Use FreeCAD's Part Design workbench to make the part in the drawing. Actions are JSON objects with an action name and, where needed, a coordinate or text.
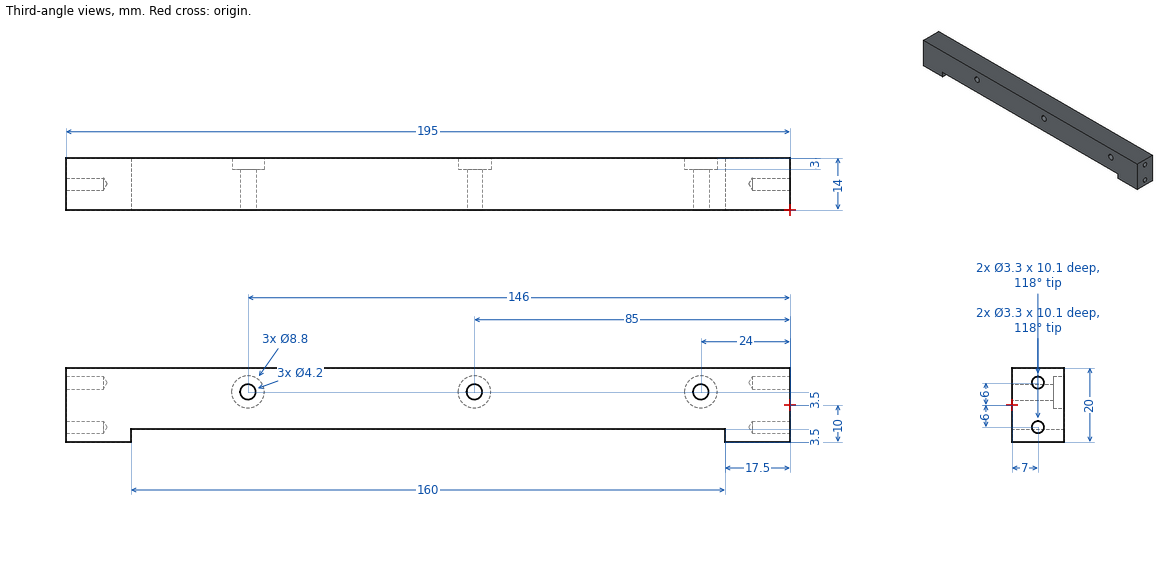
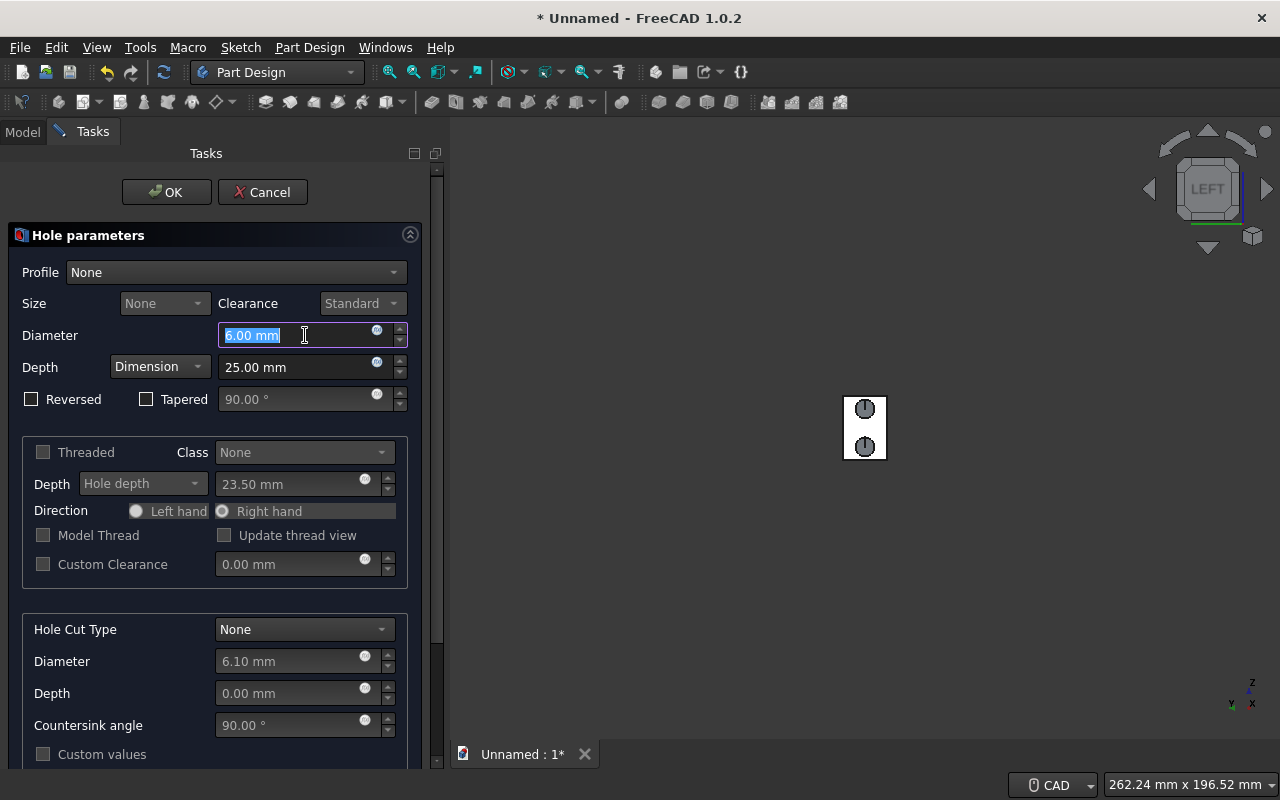
{"action": "type", "text": "3.3"}
{"action": "key", "text": "Tab"}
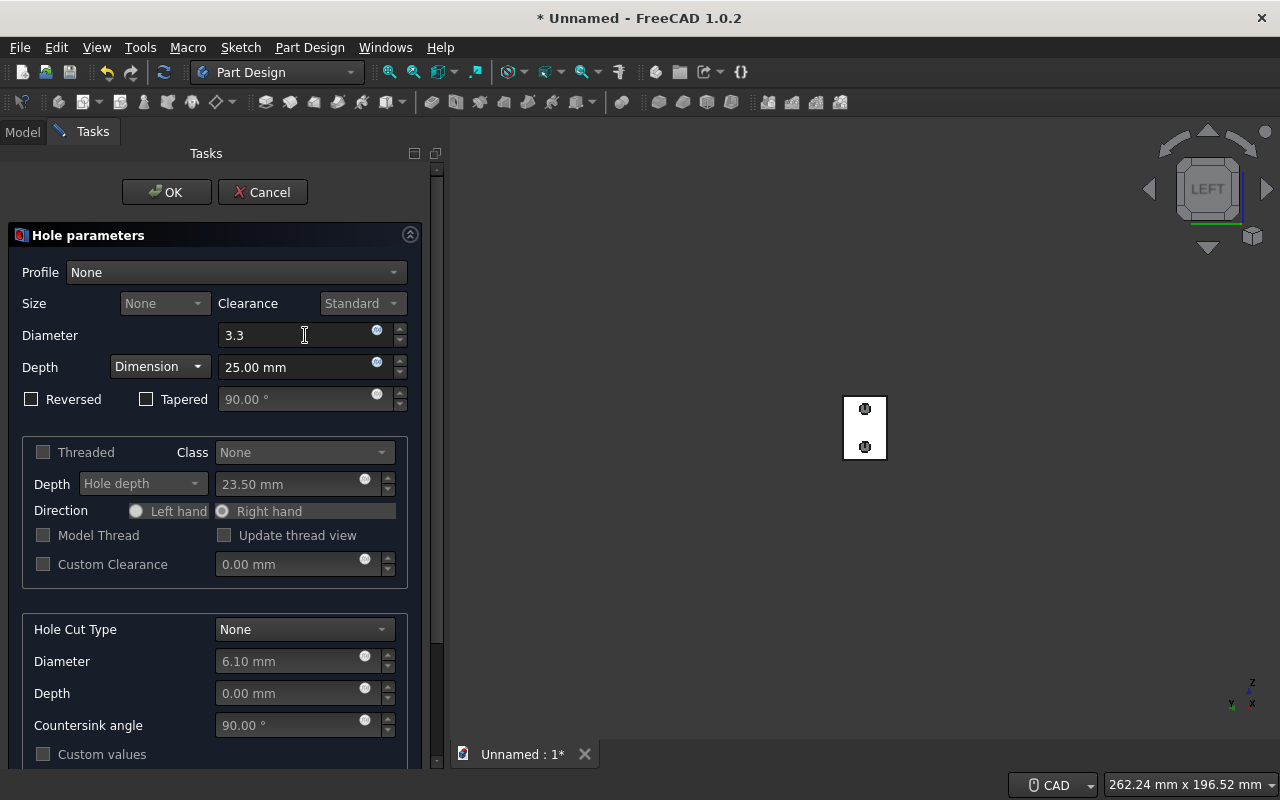
{"action": "triple_click", "coordinate": [305, 367]}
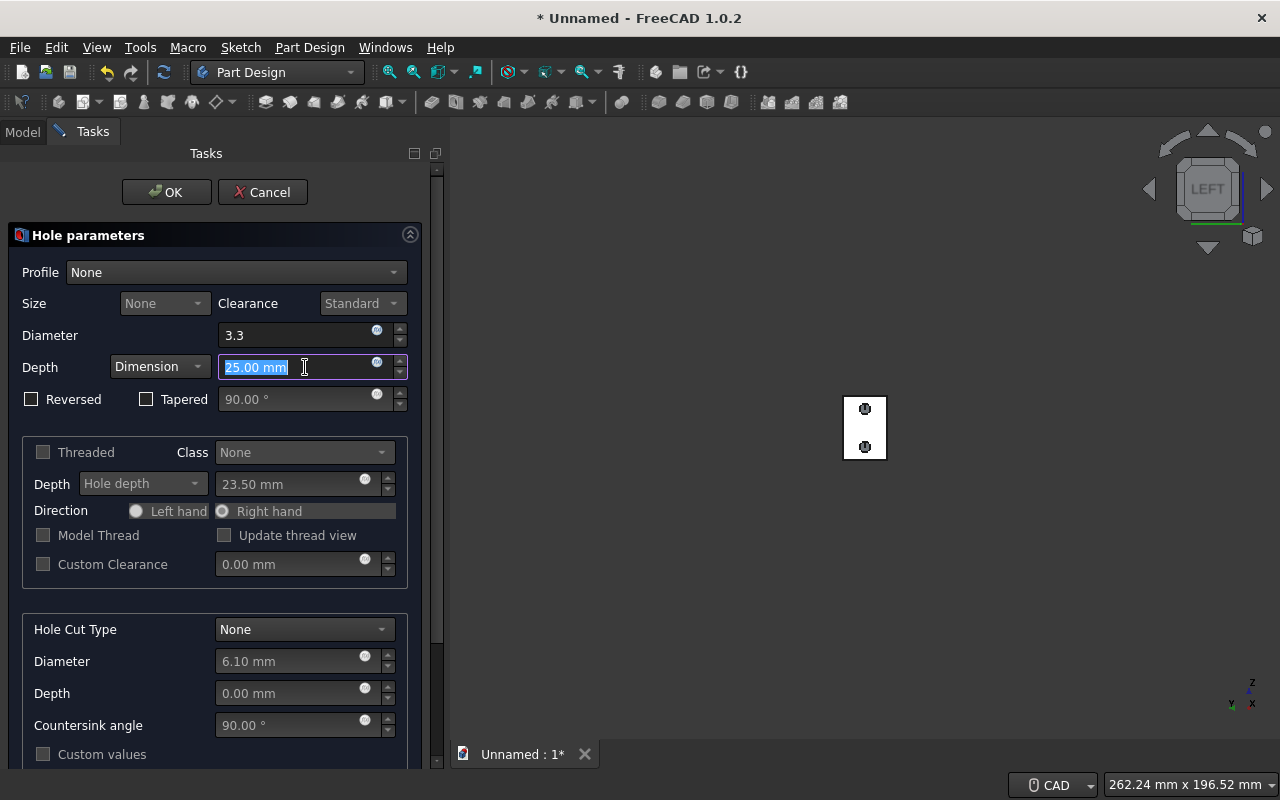
{"action": "type", "text": "10.1"}
{"action": "key", "text": "Tab"}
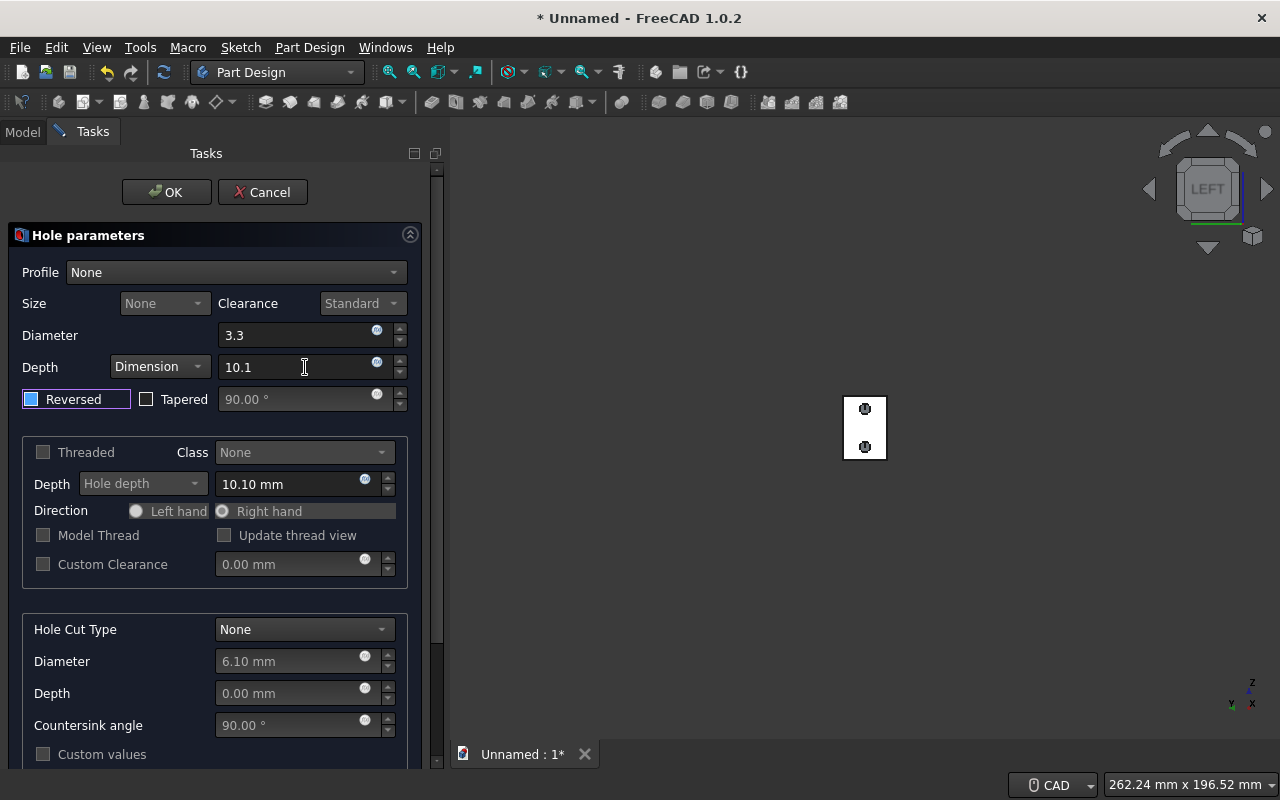
{"action": "left_click", "coordinate": [167, 192]}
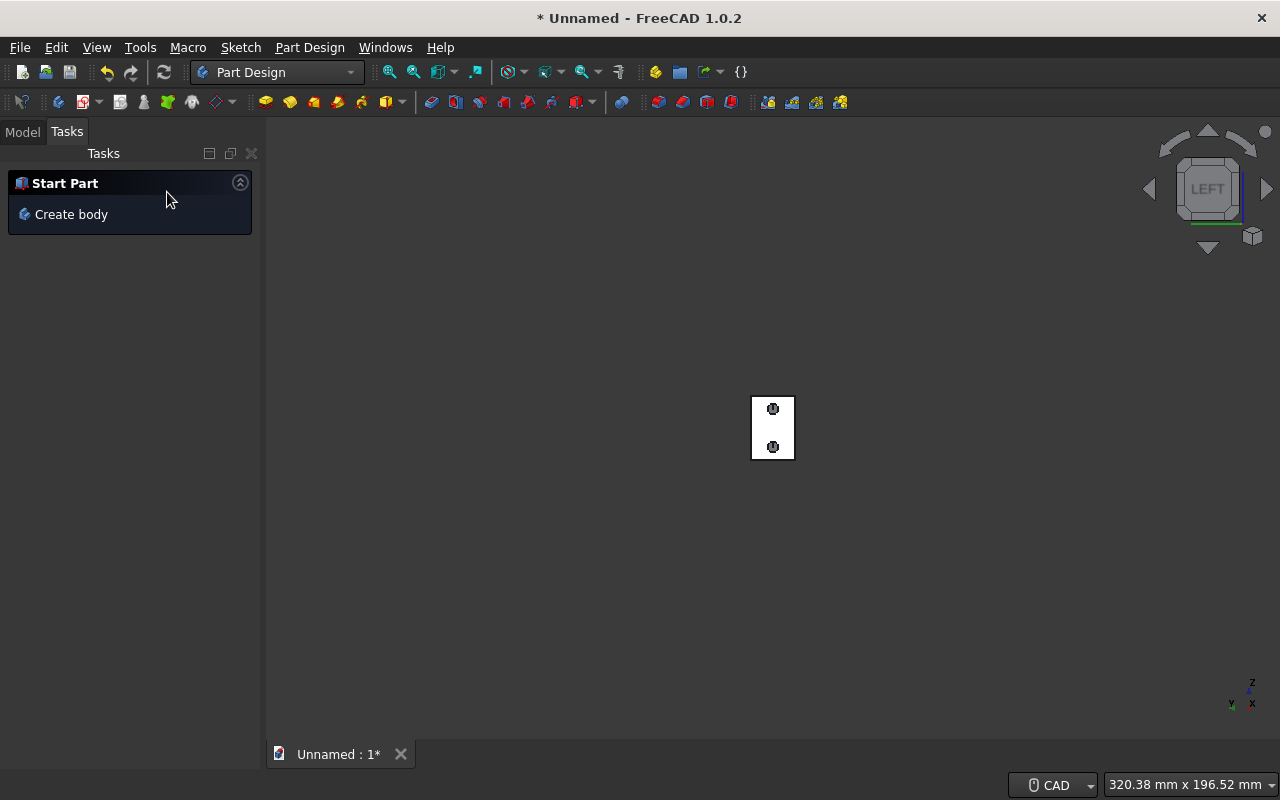
{"action": "key", "text": "v f"}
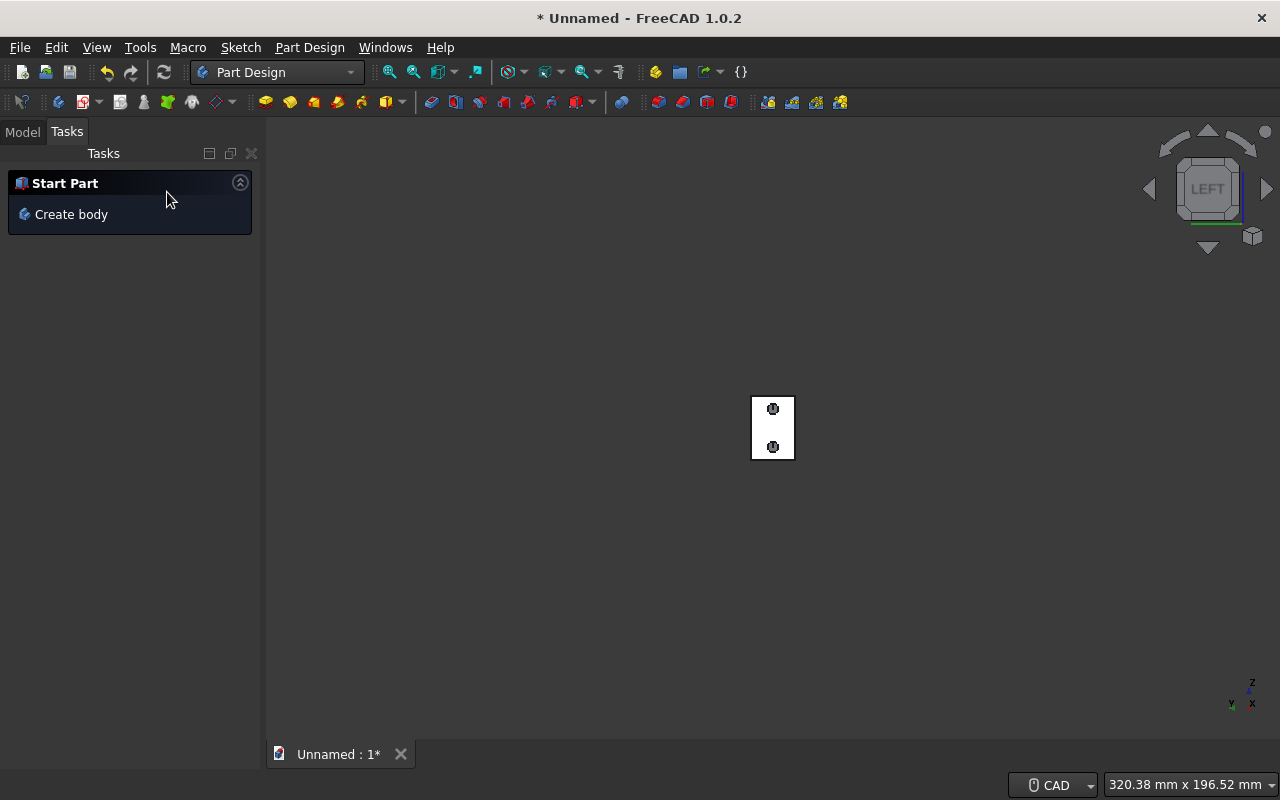
{"action": "key", "text": "0"}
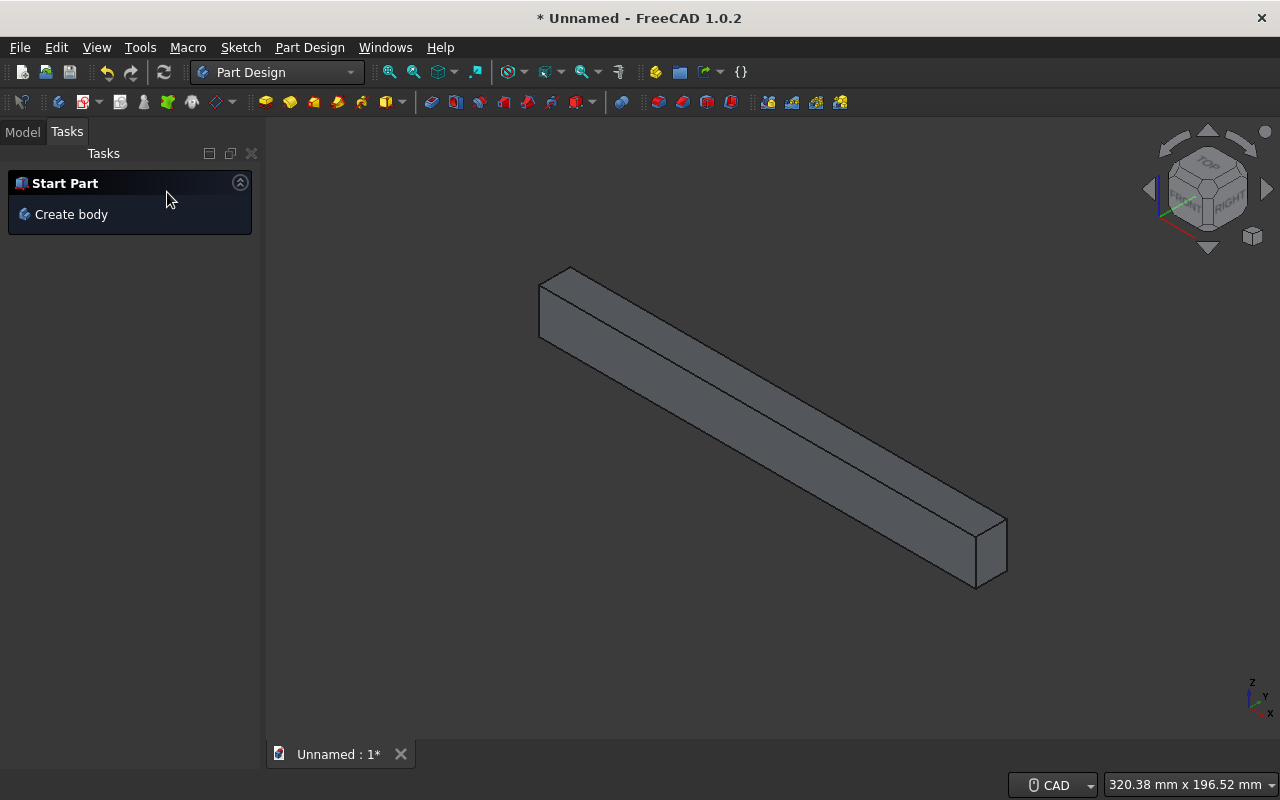
{"action": "left_click", "coordinate": [991, 546]}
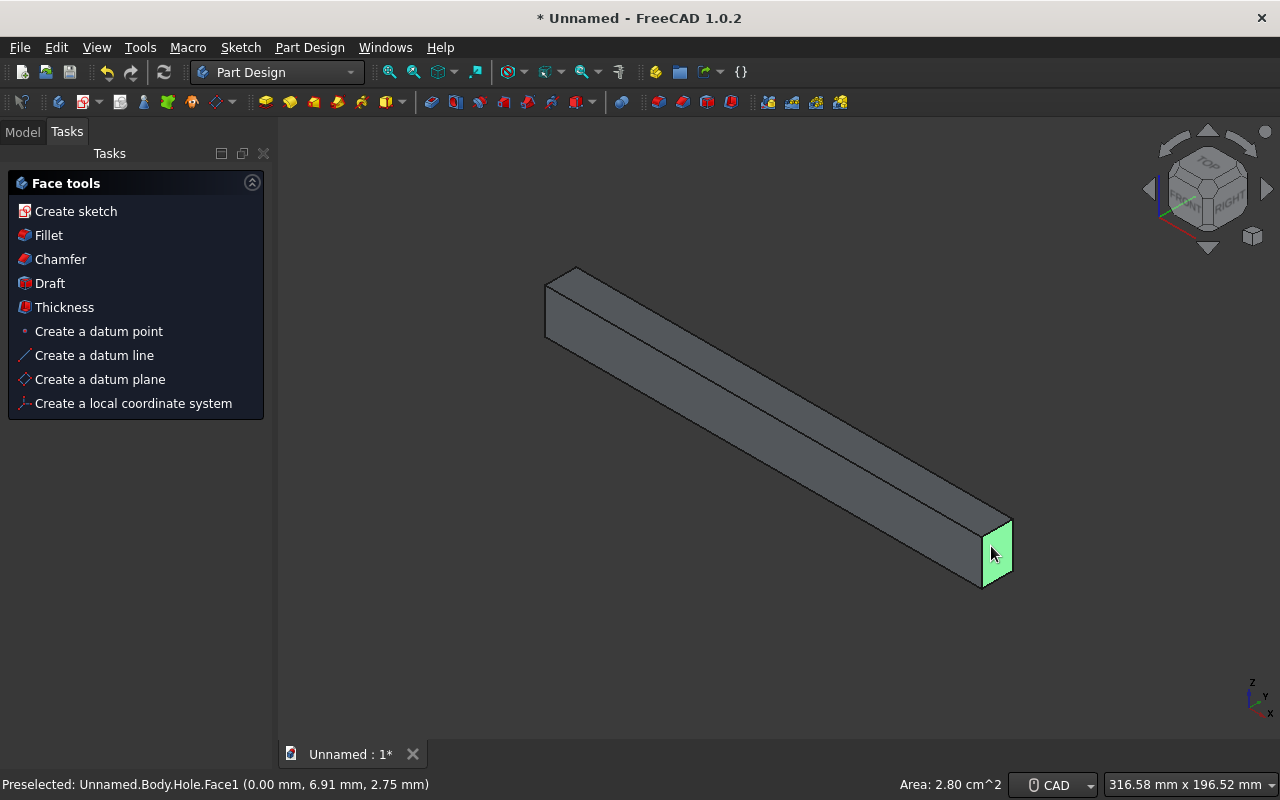
{"action": "left_click", "coordinate": [84, 102]}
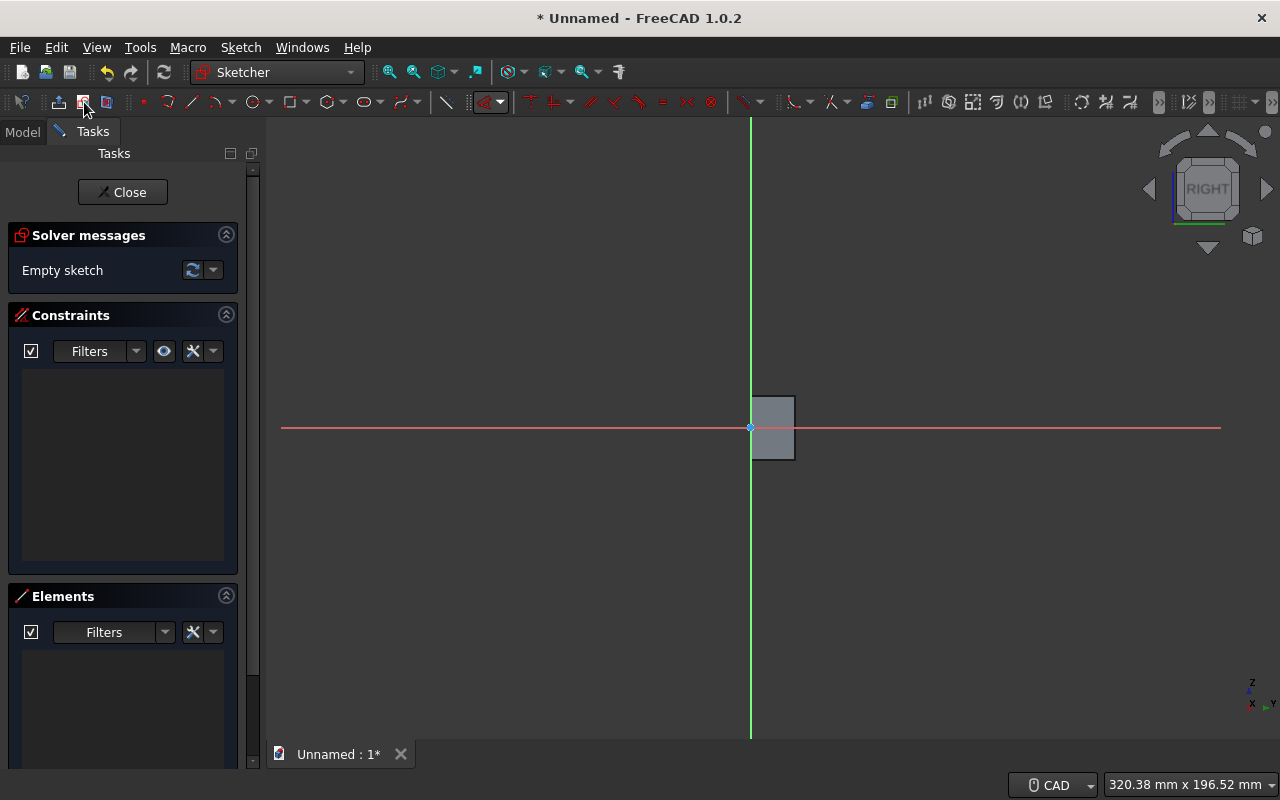
{"action": "scroll", "coordinate": [772, 428], "scroll_direction": "up", "scroll_amount": 11}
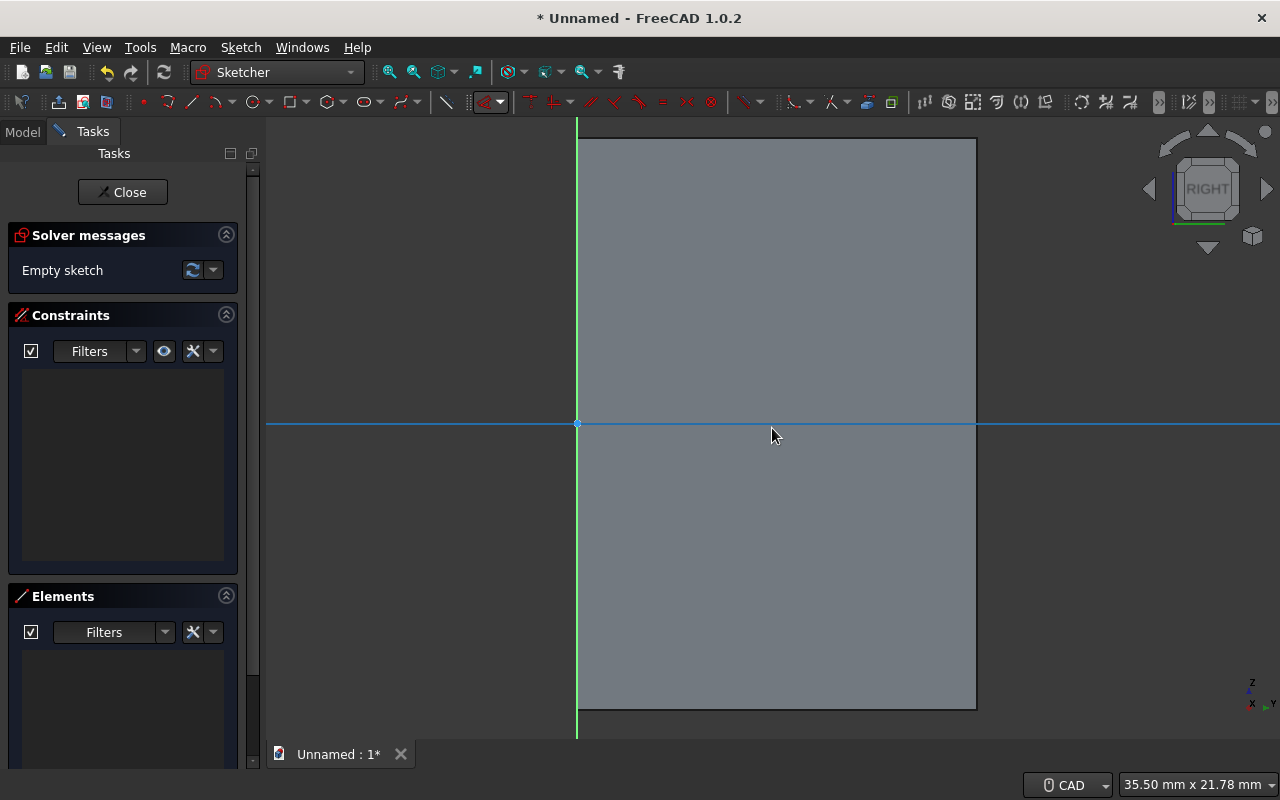
{"action": "left_click", "coordinate": [254, 102]}